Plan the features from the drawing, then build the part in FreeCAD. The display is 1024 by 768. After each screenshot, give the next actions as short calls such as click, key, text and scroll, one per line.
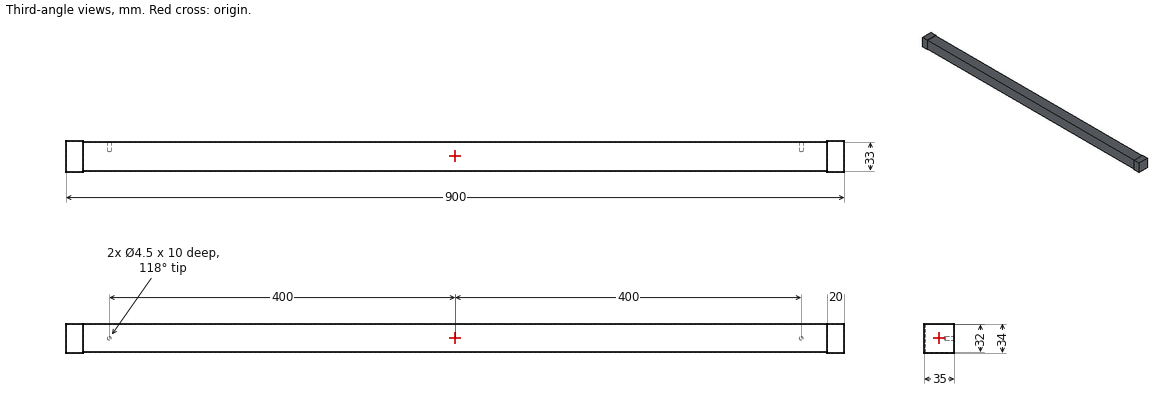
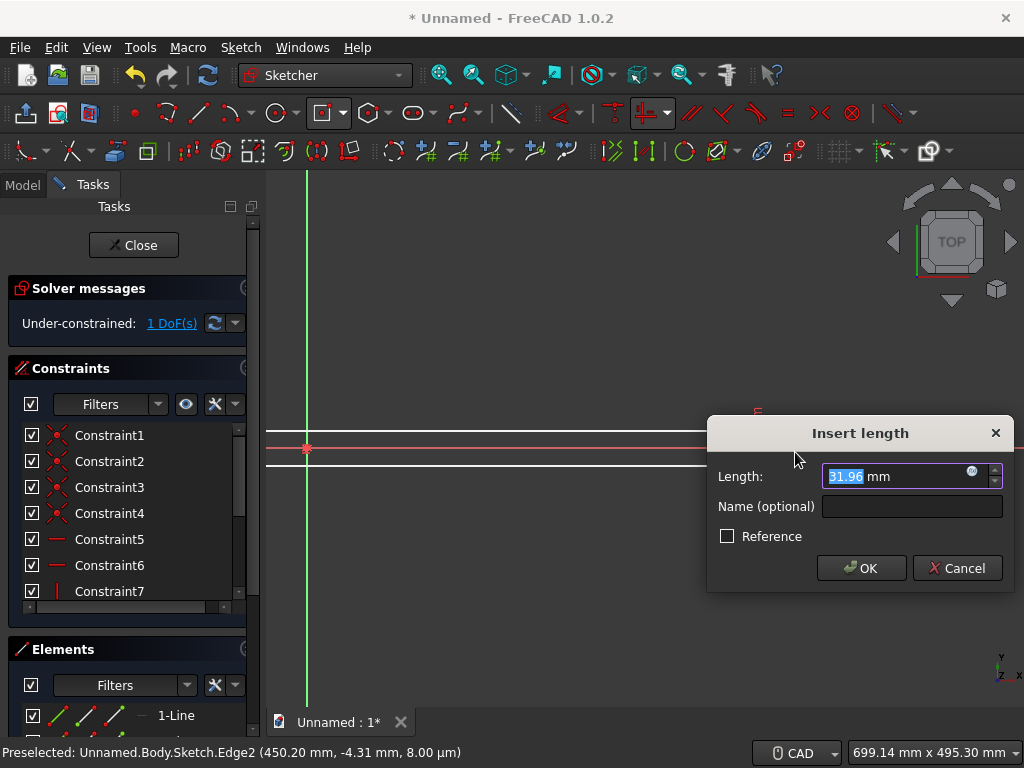
text(33)
key(Return)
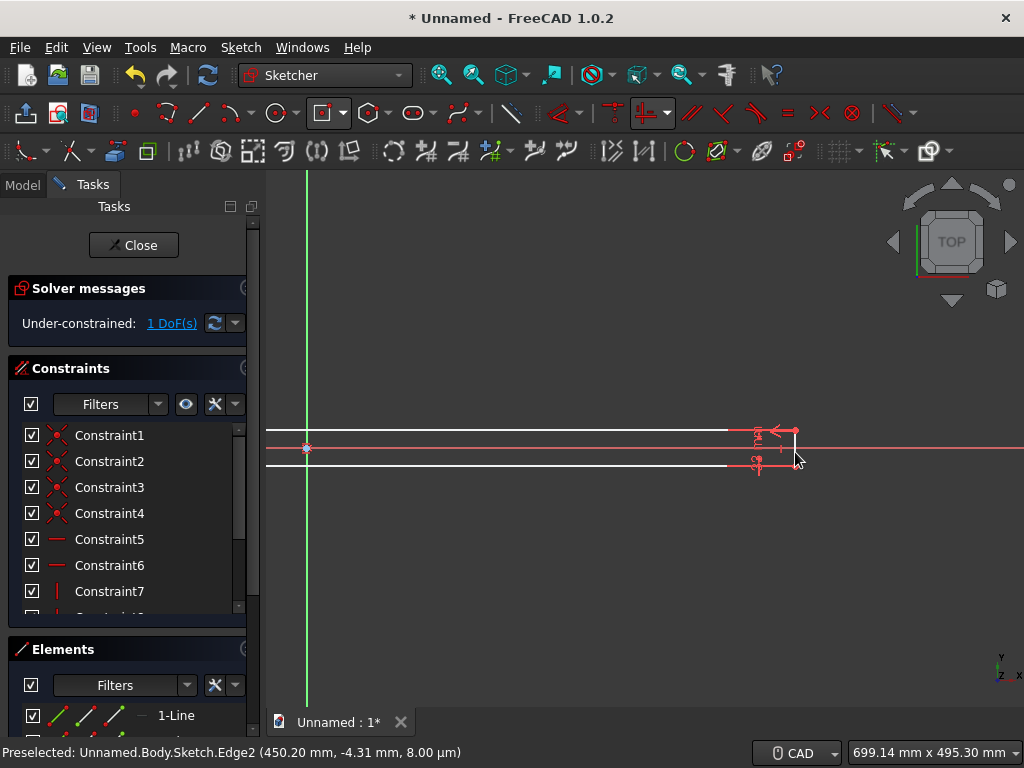
click(502, 466)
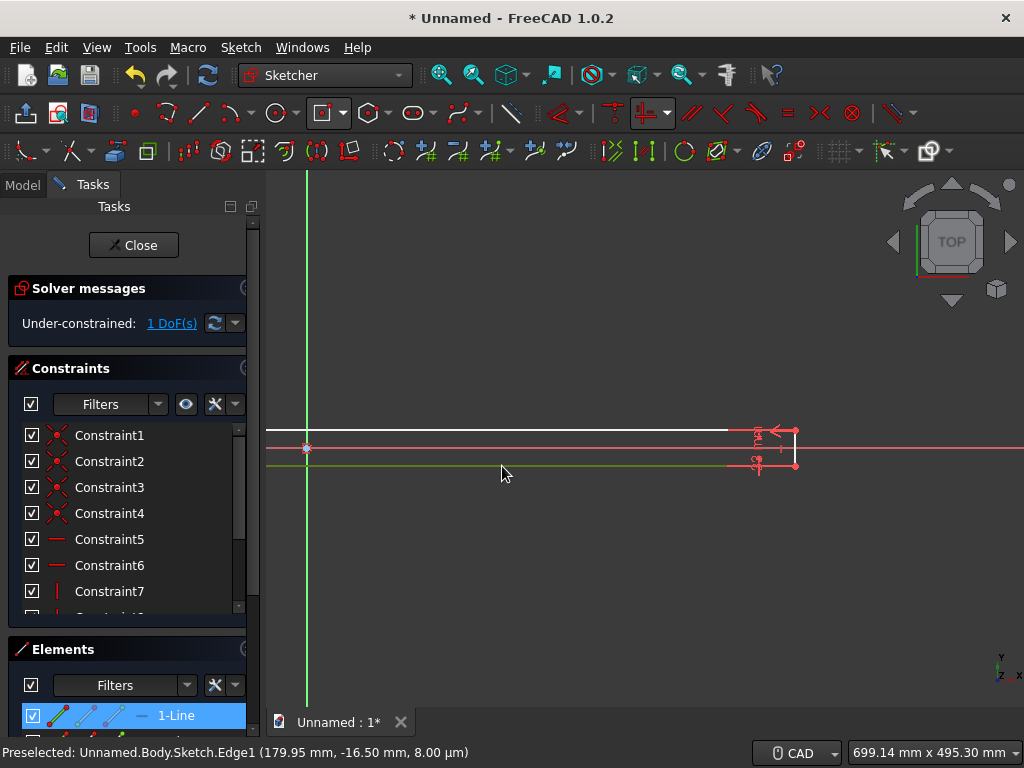
key(l)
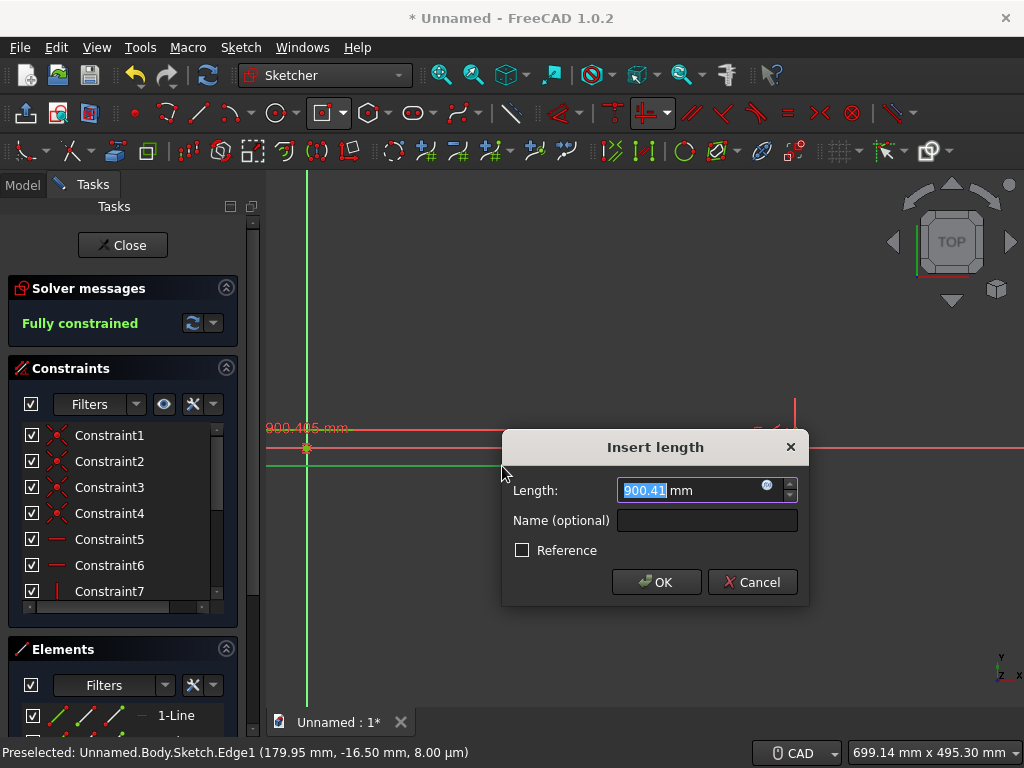
text(900)
key(Return)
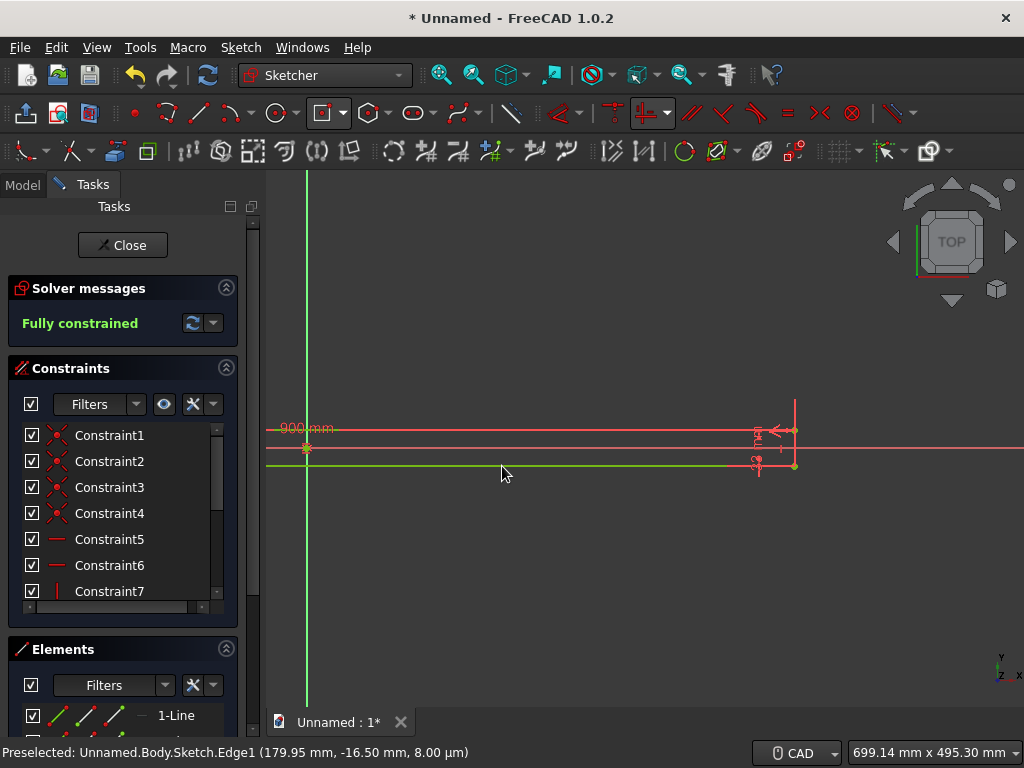
click(123, 245)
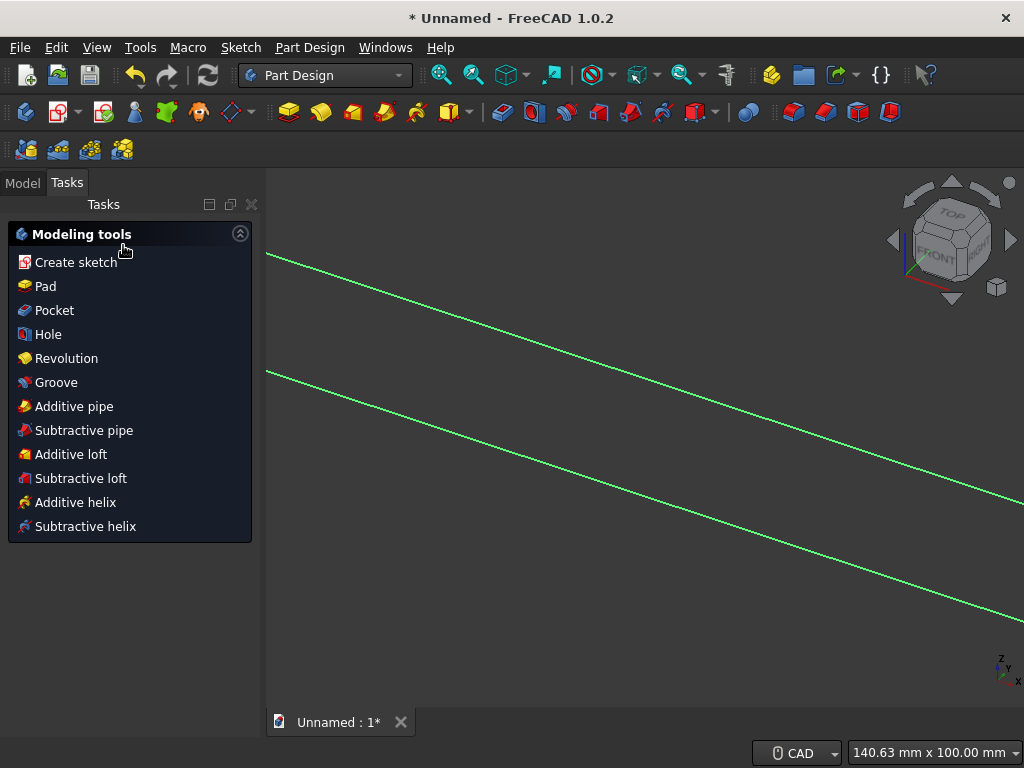
click(290, 112)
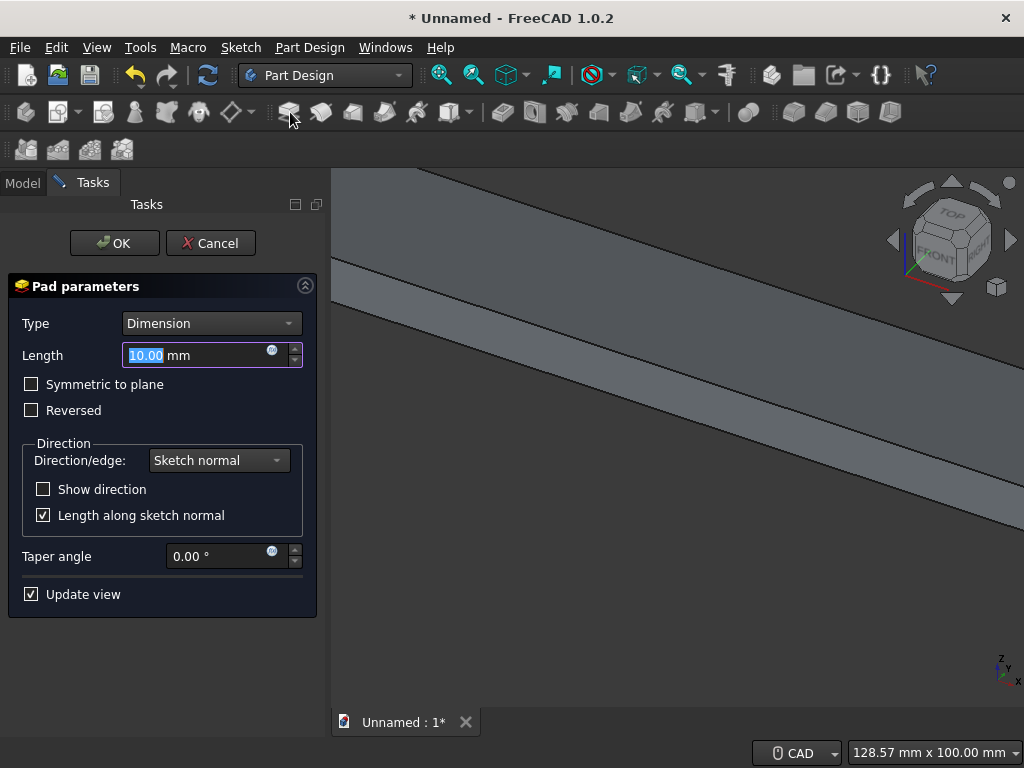
text(32)
key(Tab)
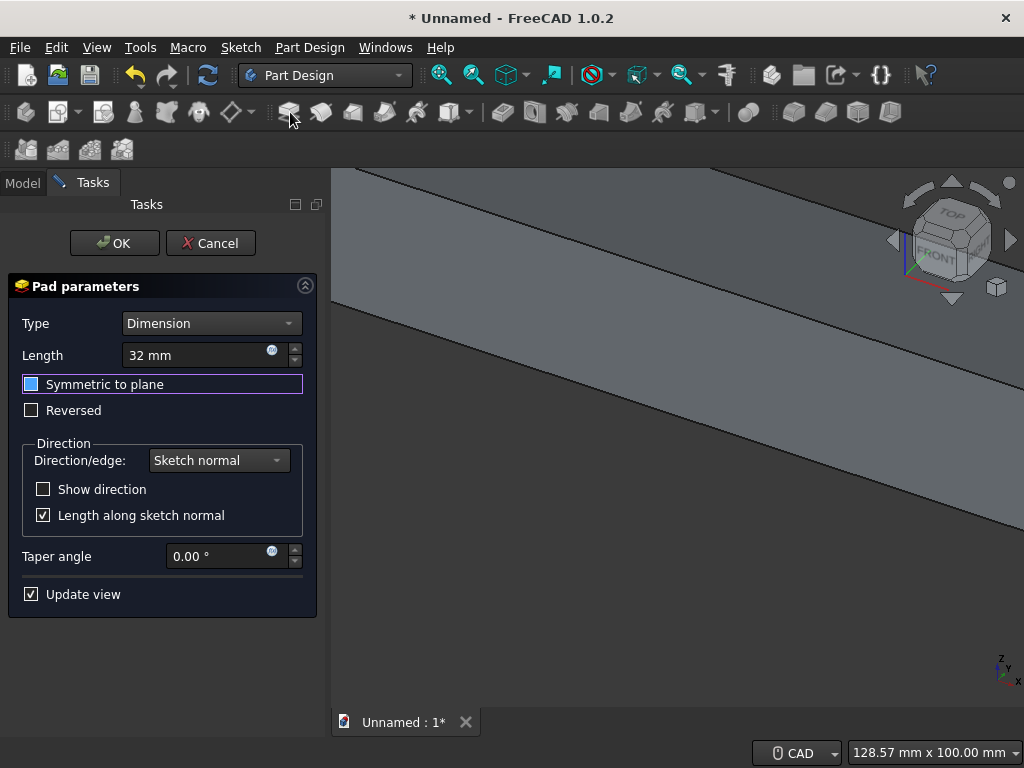
click(30, 384)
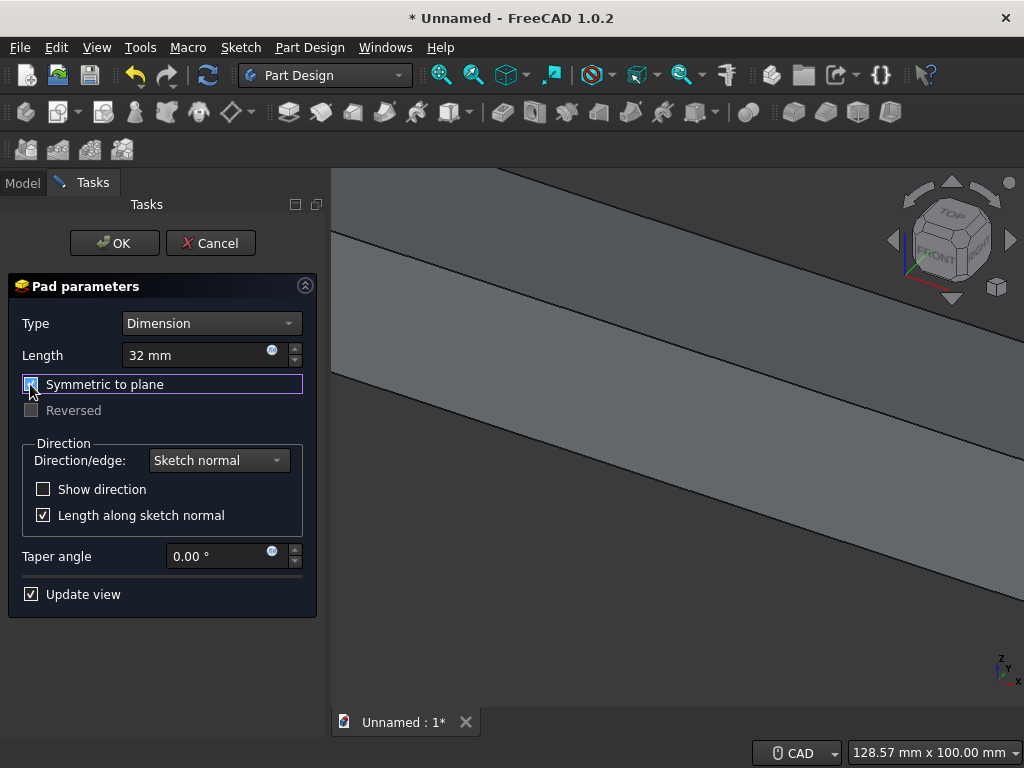
click(115, 243)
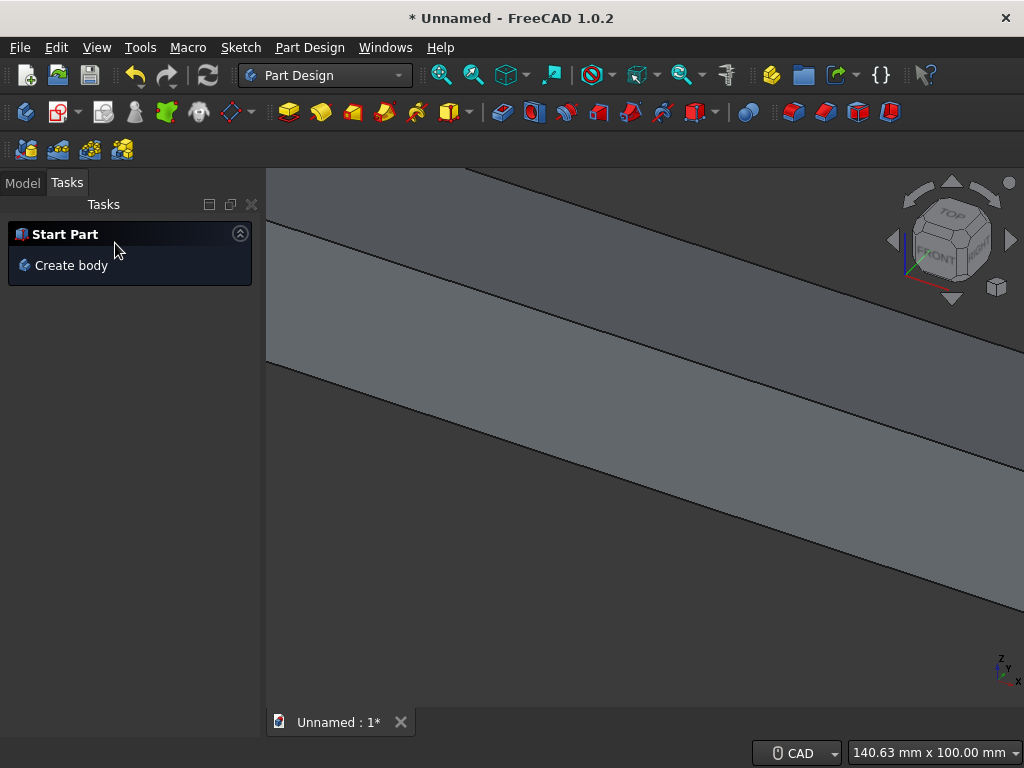
click(442, 76)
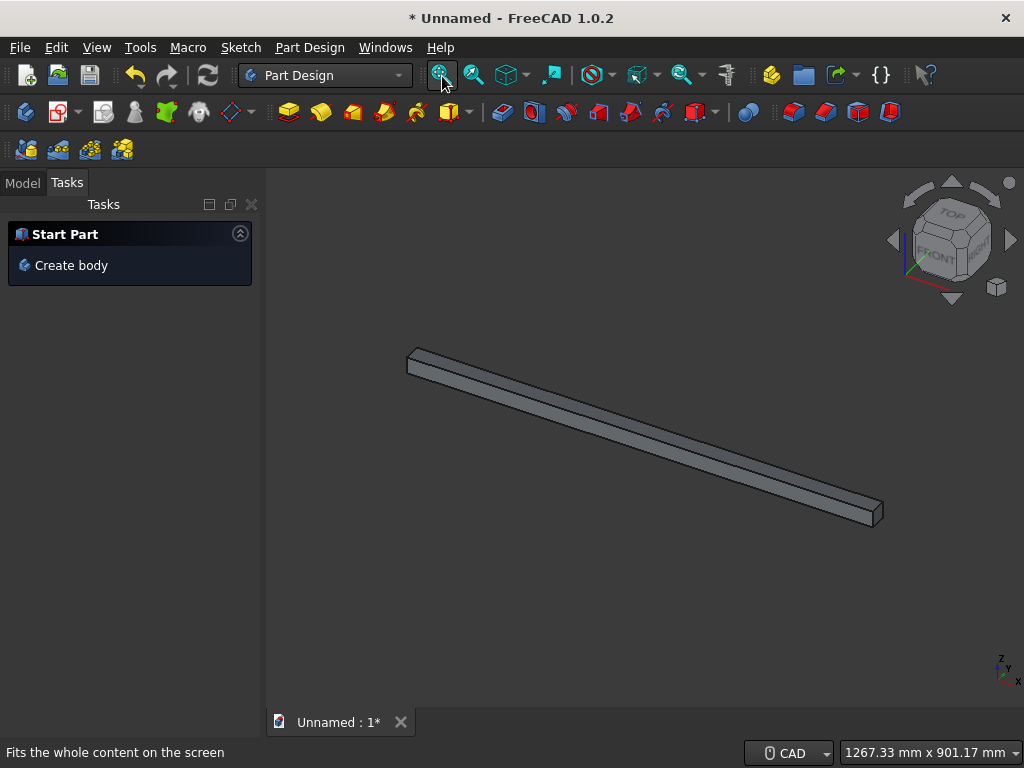
key(0)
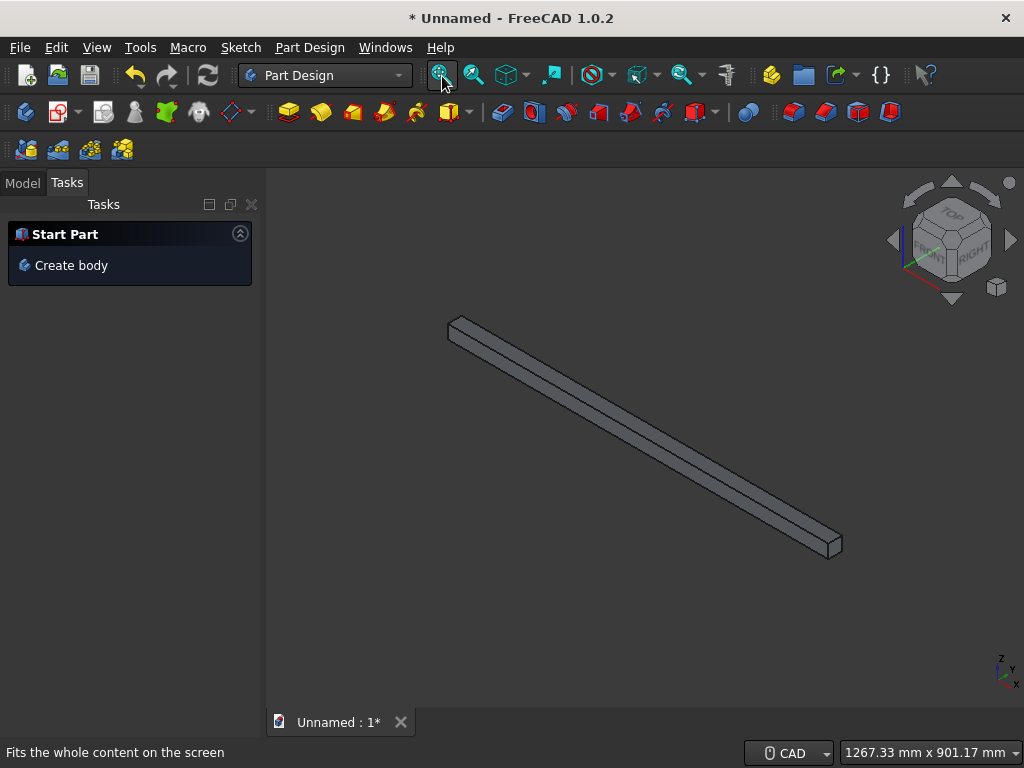
key(3)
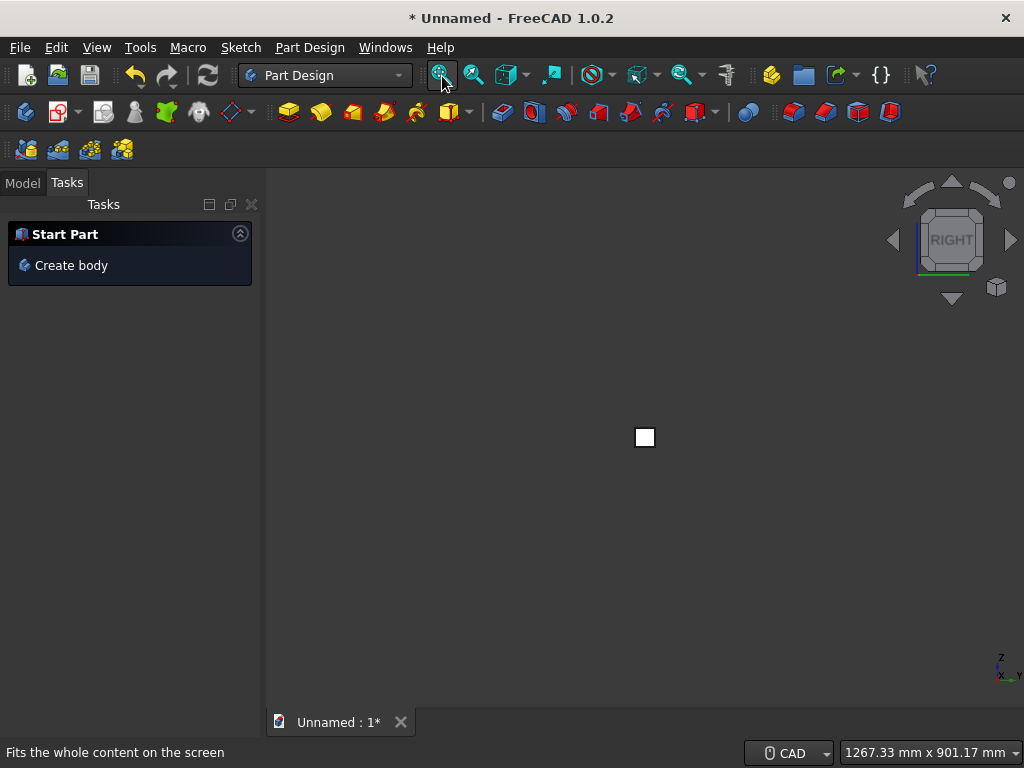
click(442, 76)